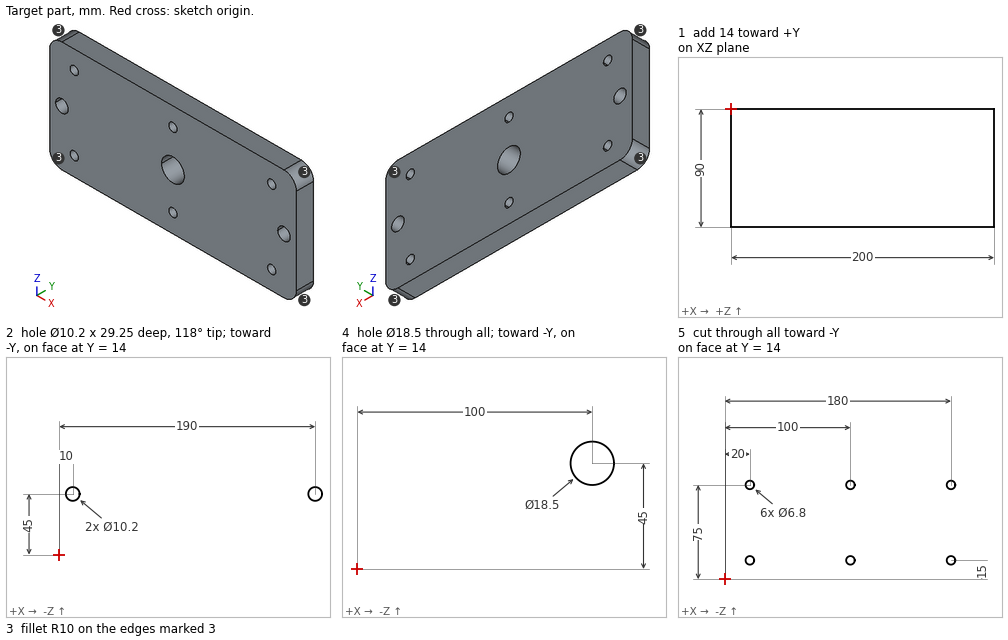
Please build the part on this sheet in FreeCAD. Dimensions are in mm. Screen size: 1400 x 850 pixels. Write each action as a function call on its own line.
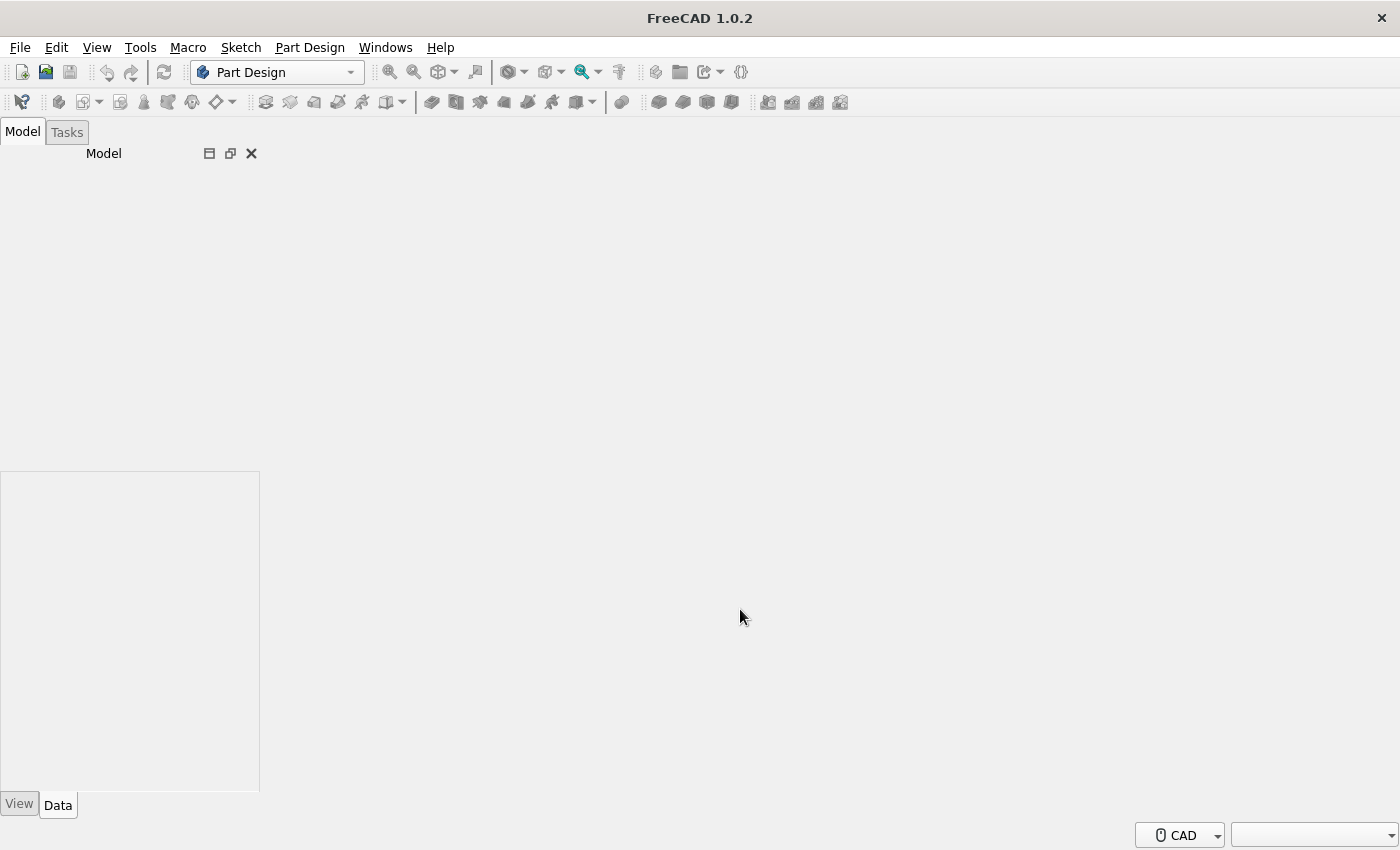
click(22, 72)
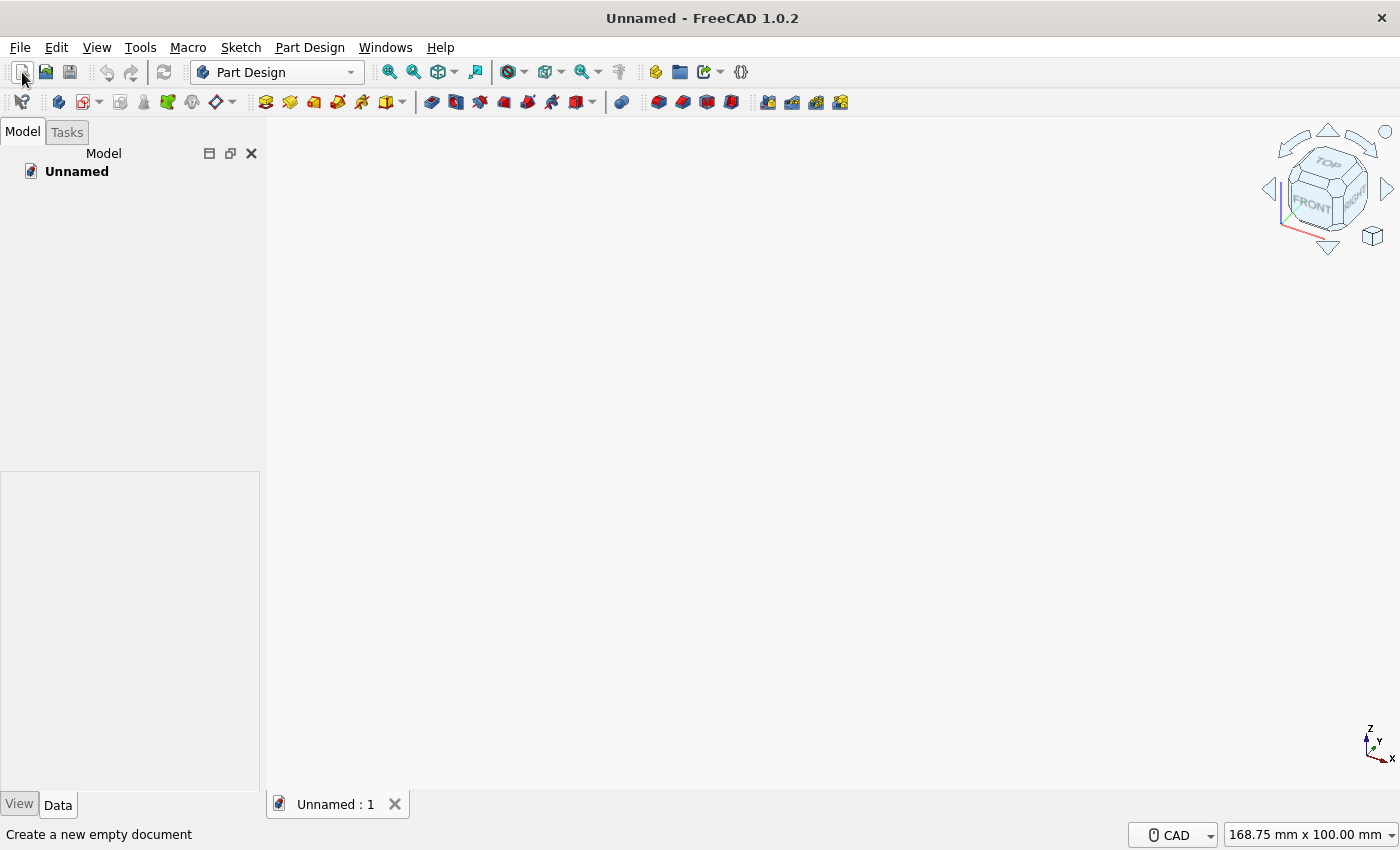
click(84, 102)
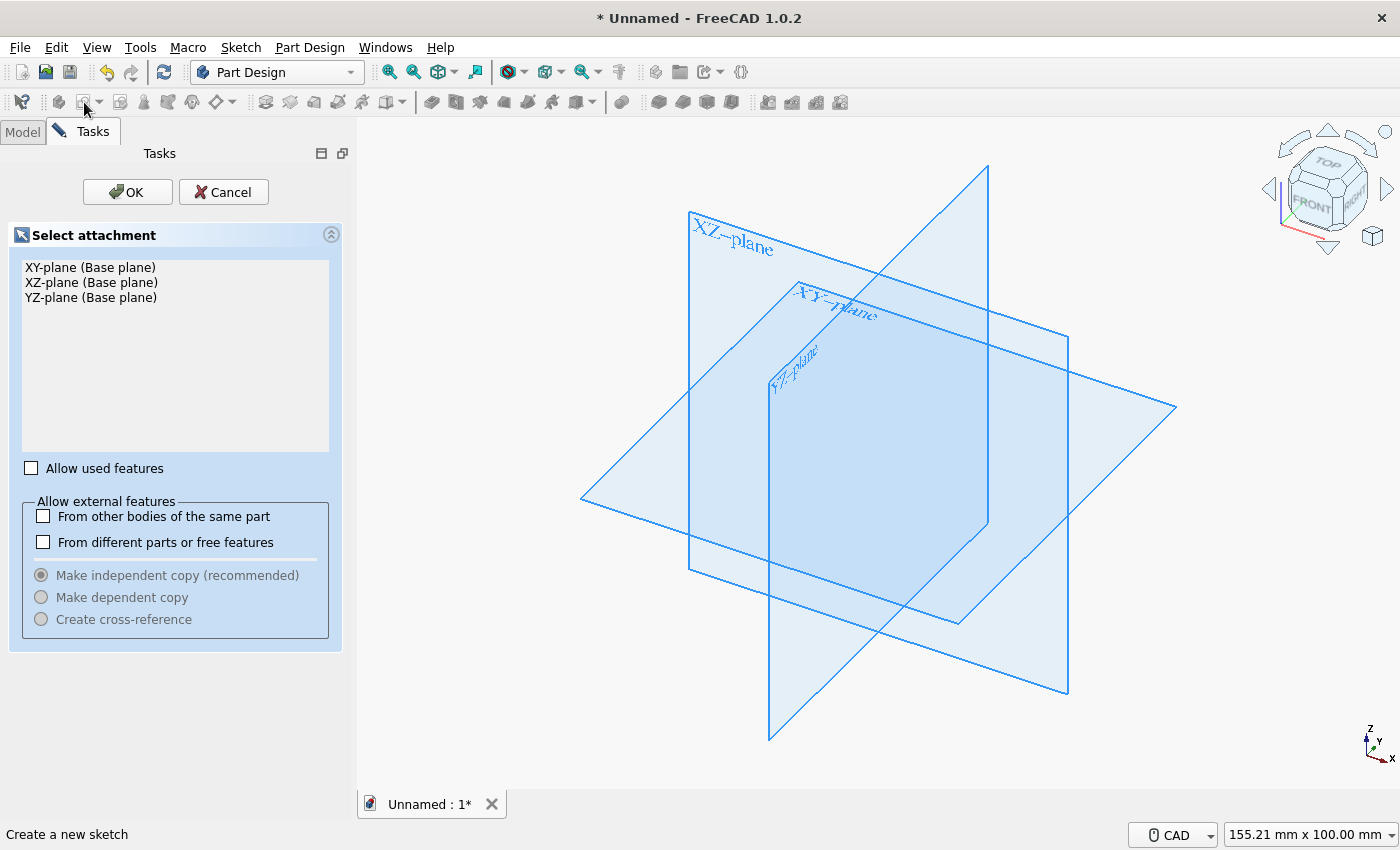
click(82, 282)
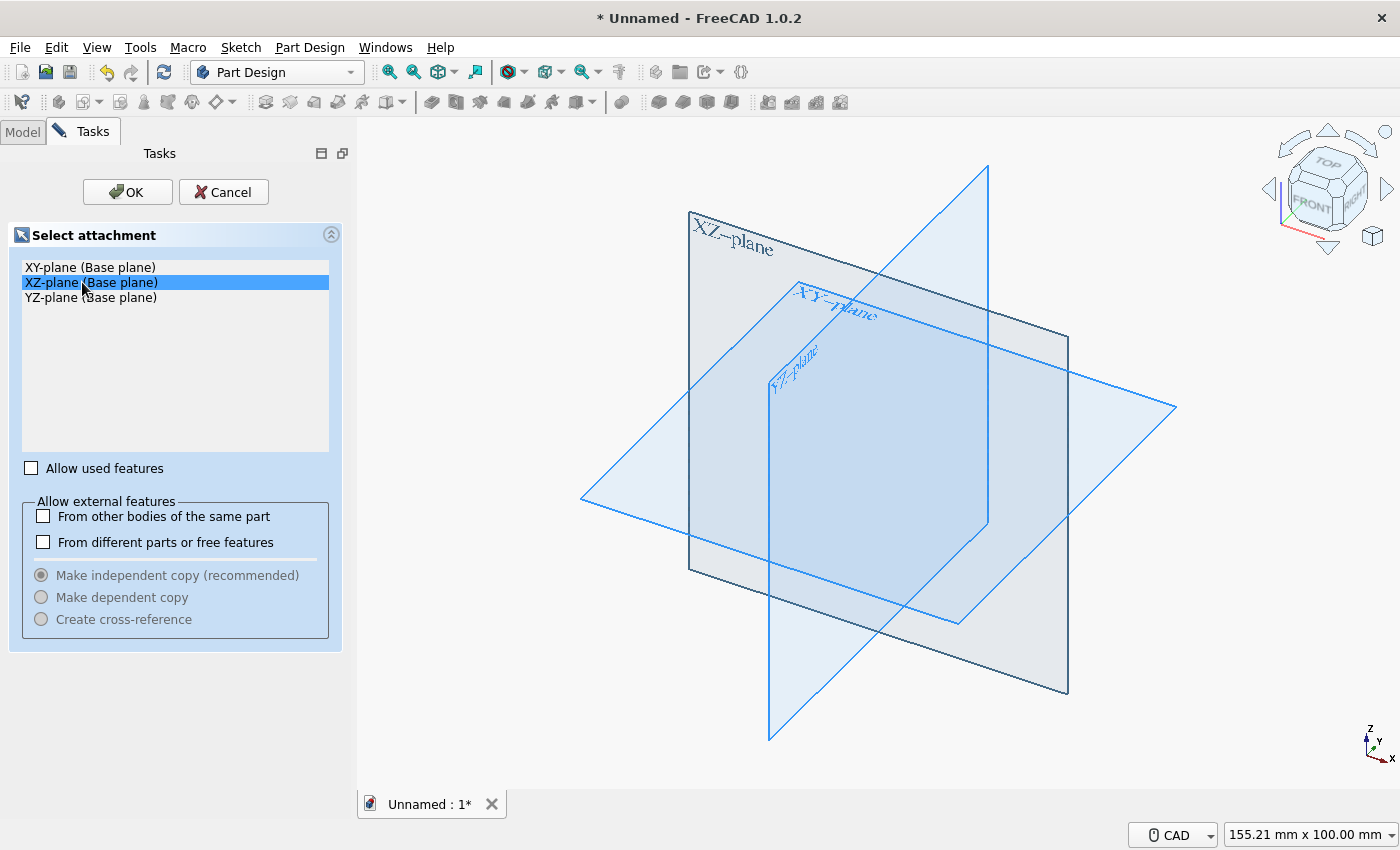
click(128, 192)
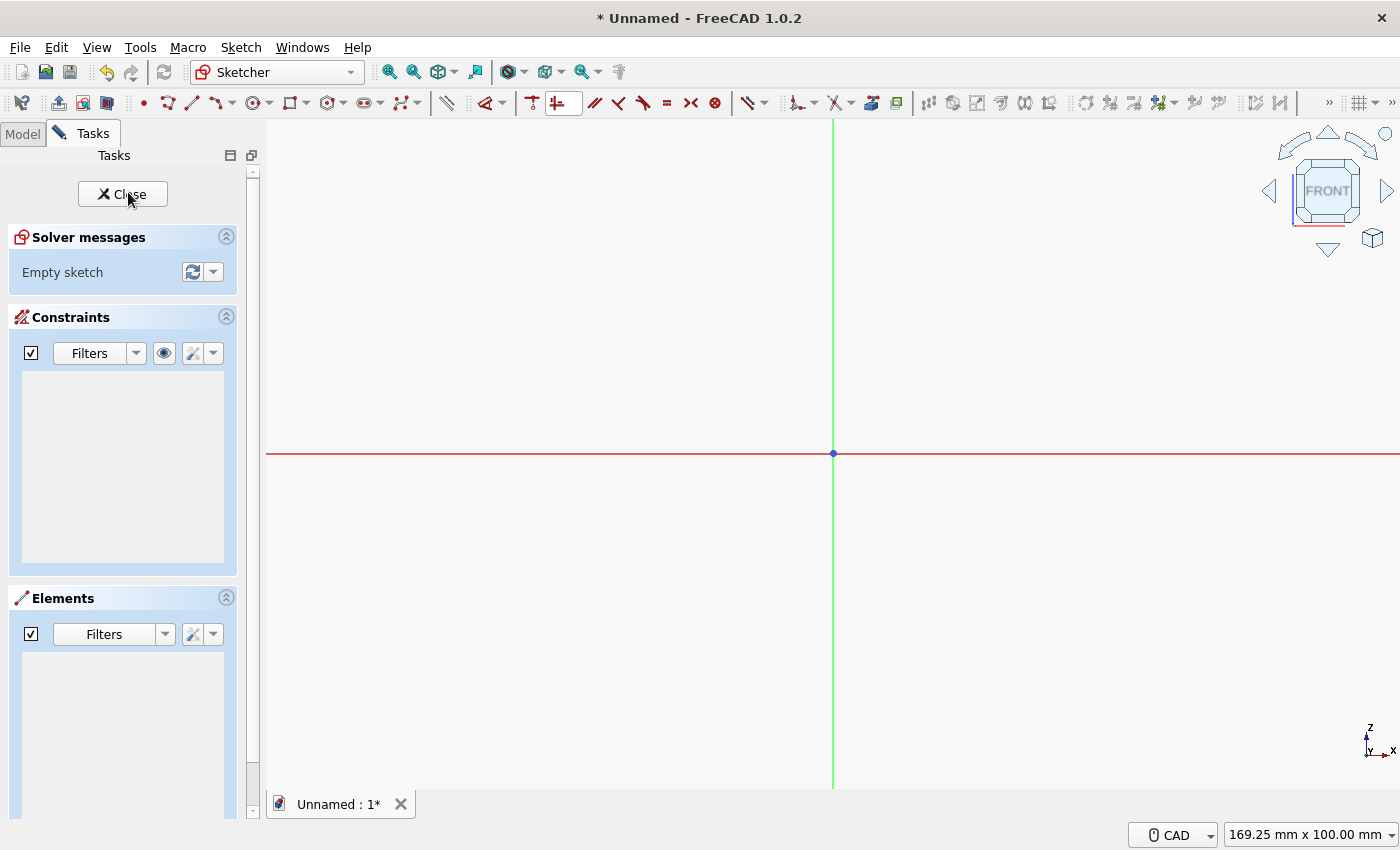
scroll(294, 208, down, 4)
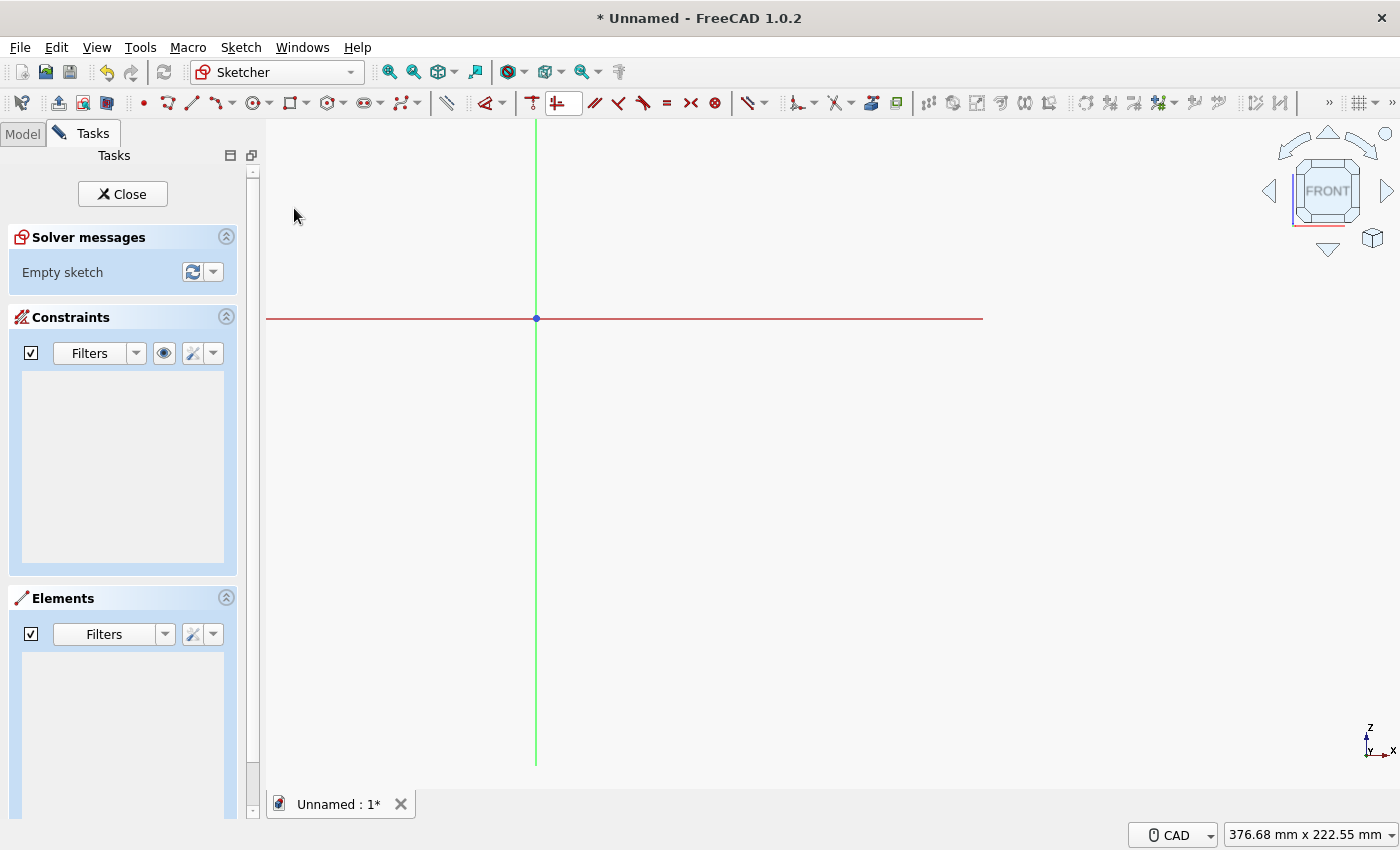
click(290, 104)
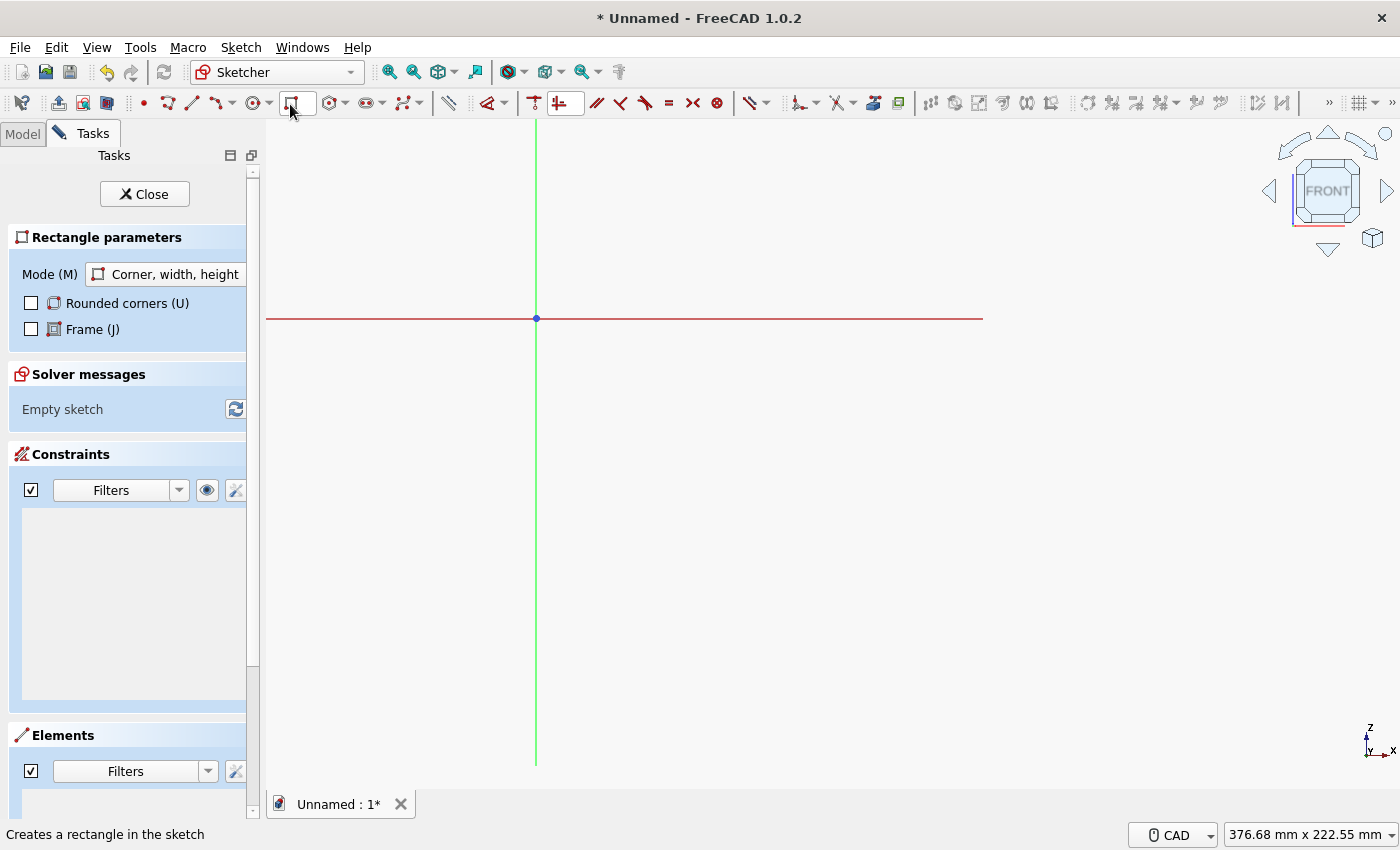
click(536, 319)
click(1138, 590)
key(Escape)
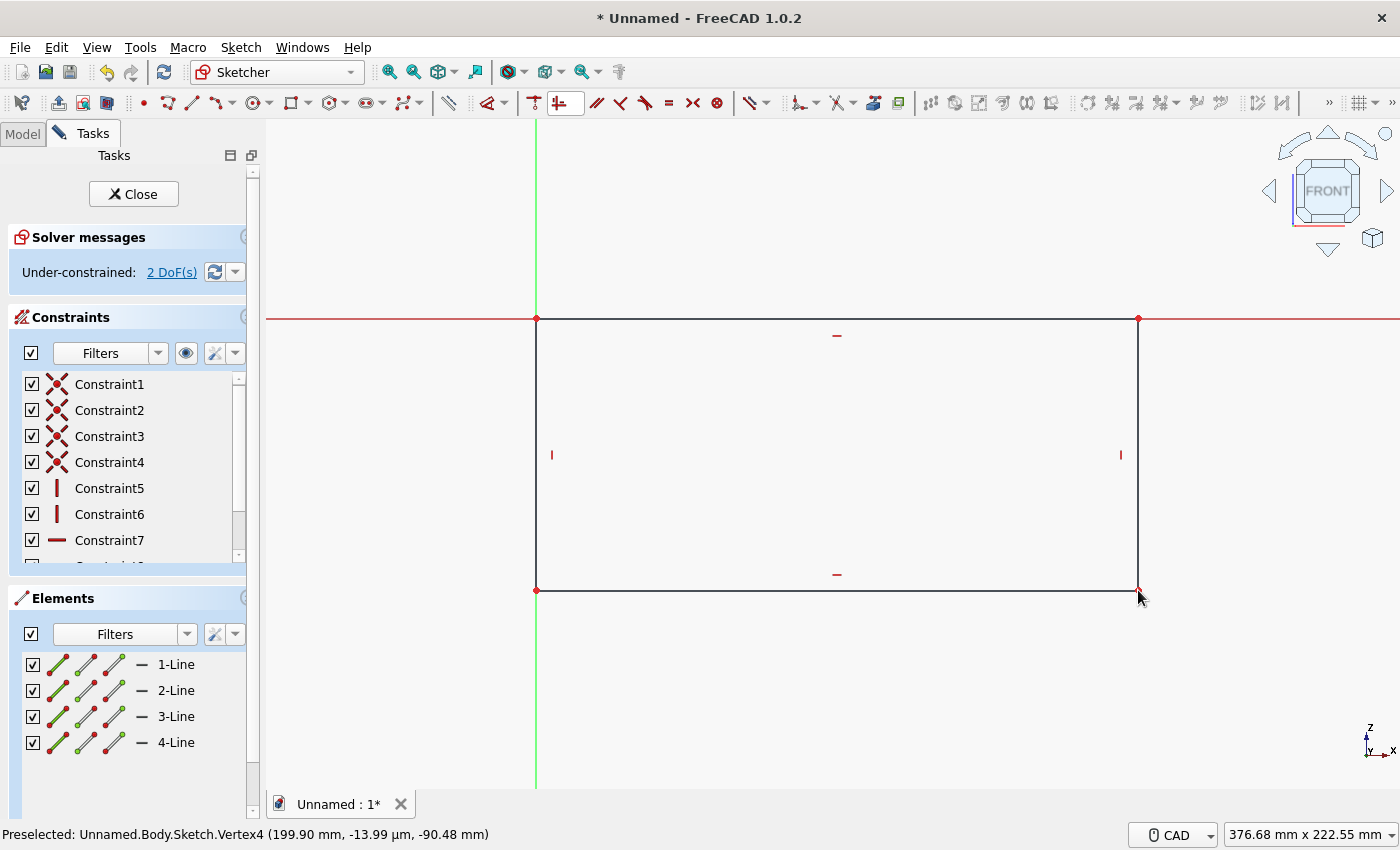
key(d)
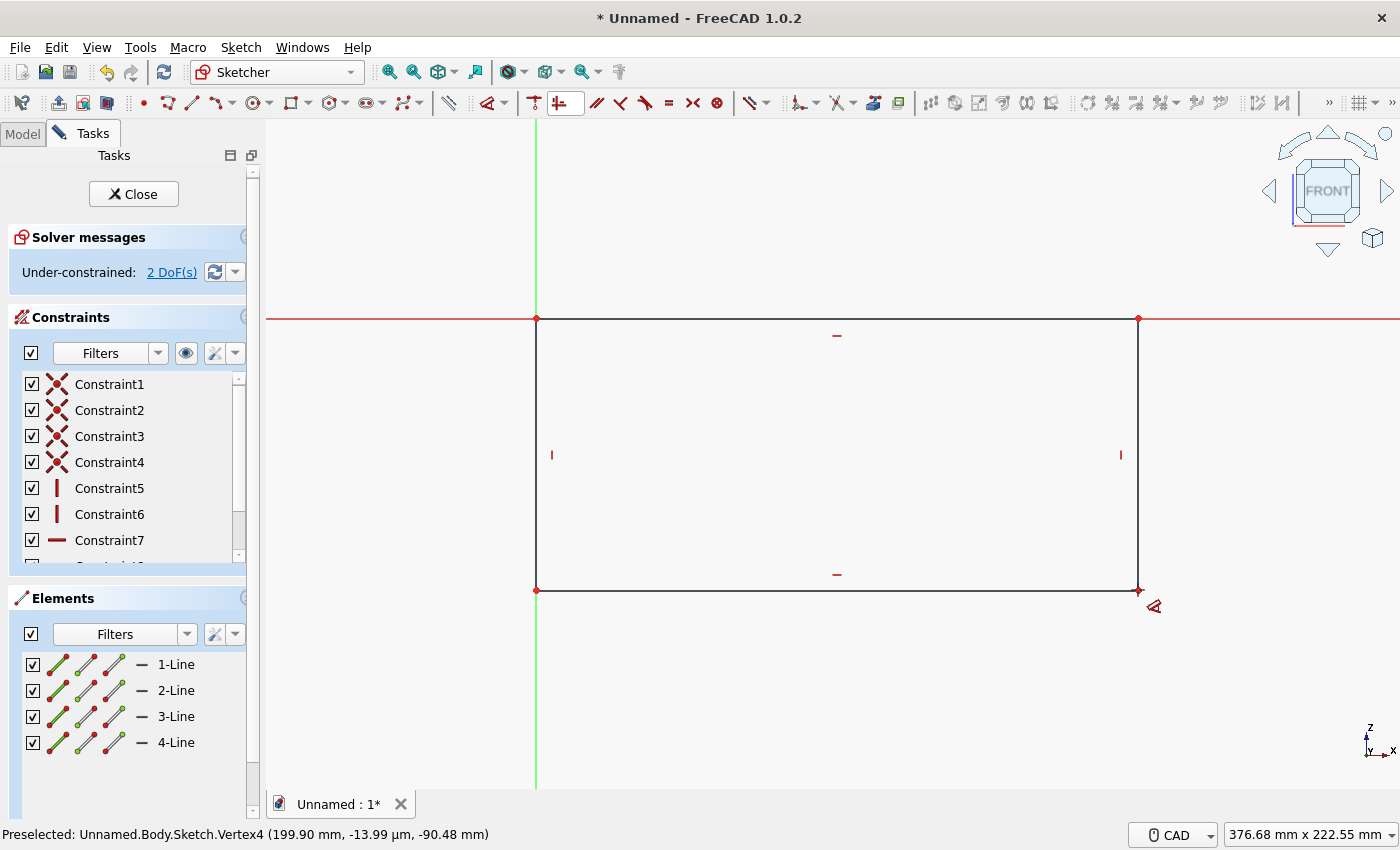
click(536, 400)
click(502, 455)